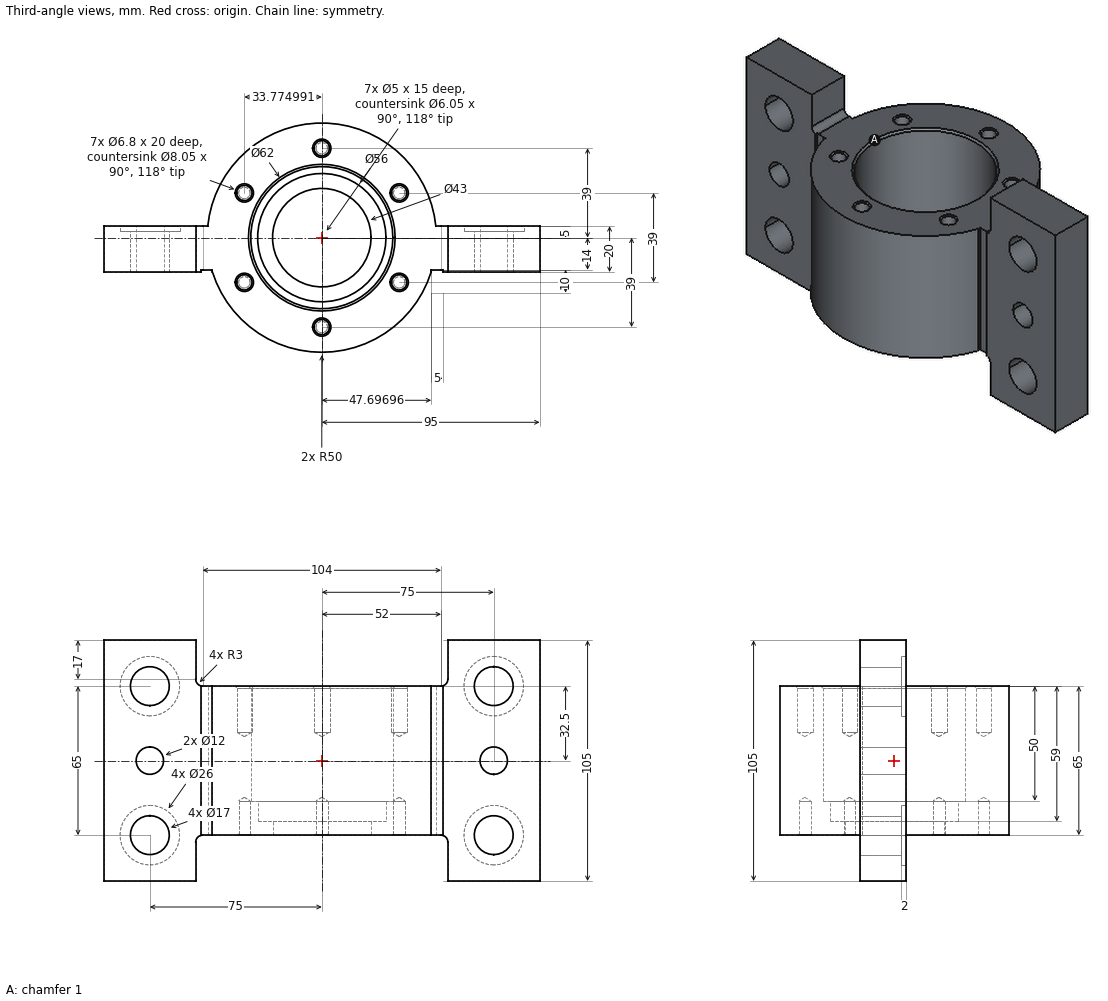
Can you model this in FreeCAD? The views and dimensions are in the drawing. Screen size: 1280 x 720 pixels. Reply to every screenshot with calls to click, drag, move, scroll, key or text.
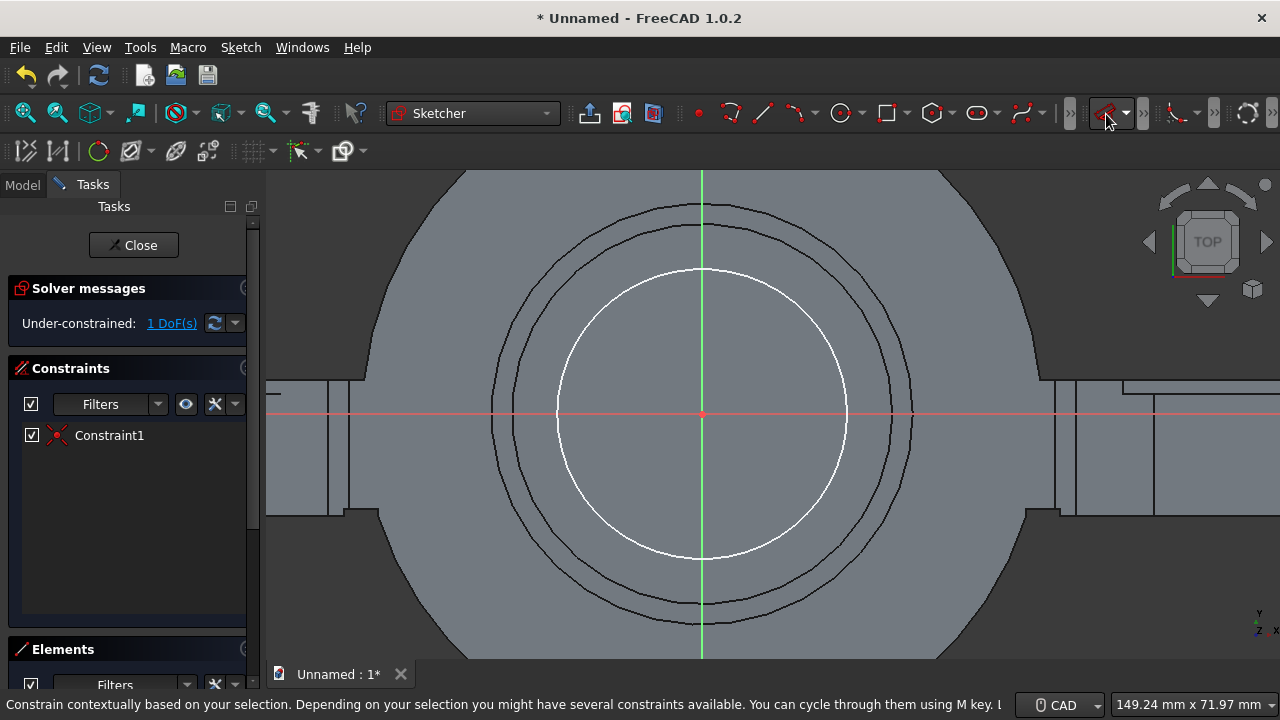
click(804, 311)
click(826, 288)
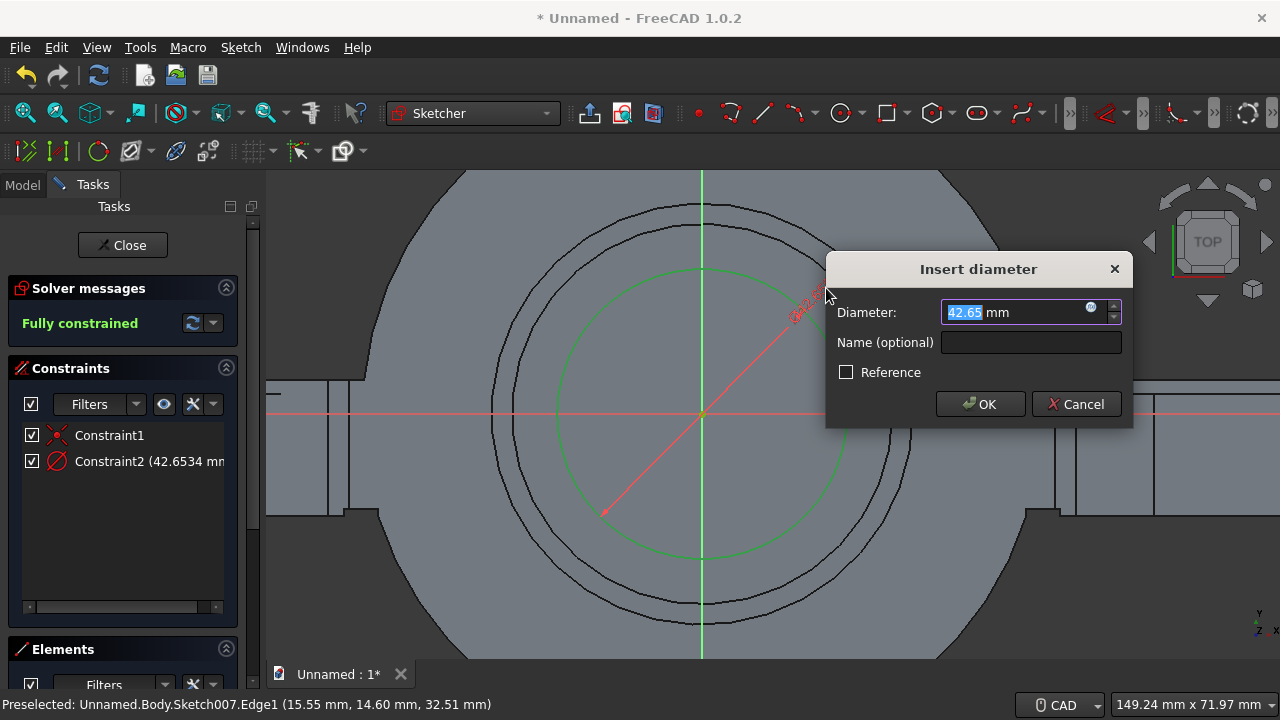
text(43)
key(Return)
key(Escape)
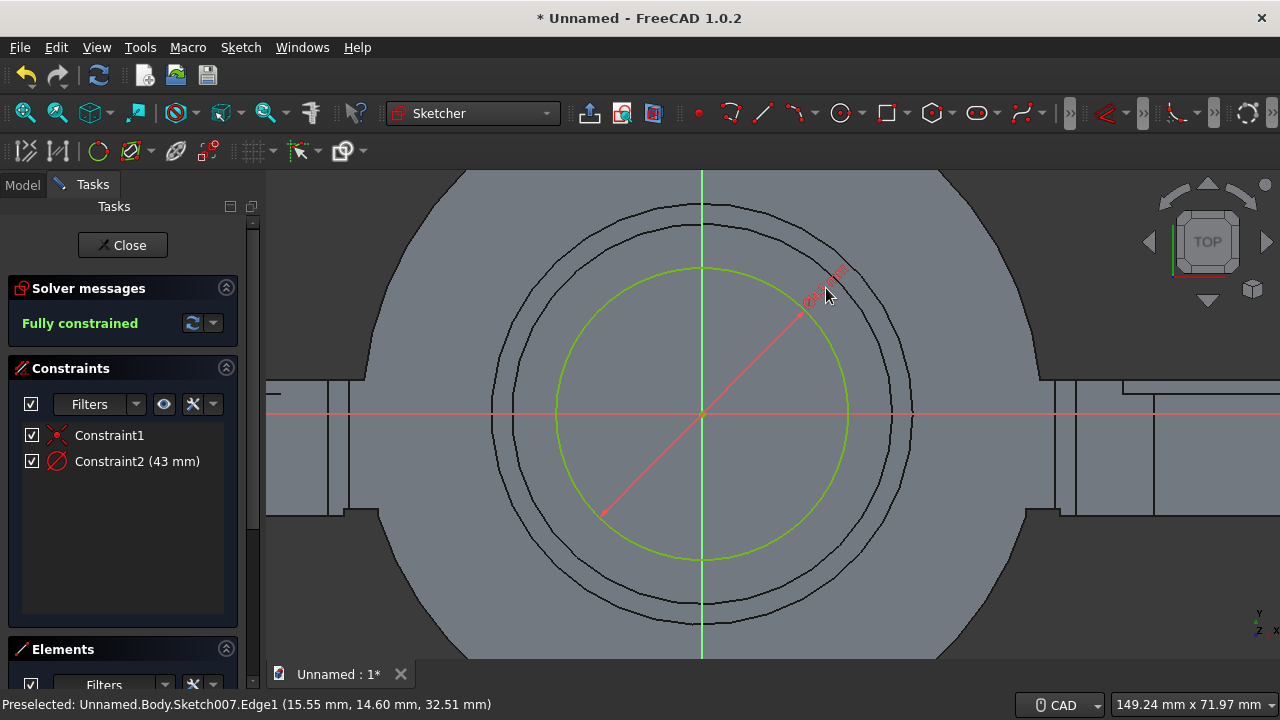
click(123, 245)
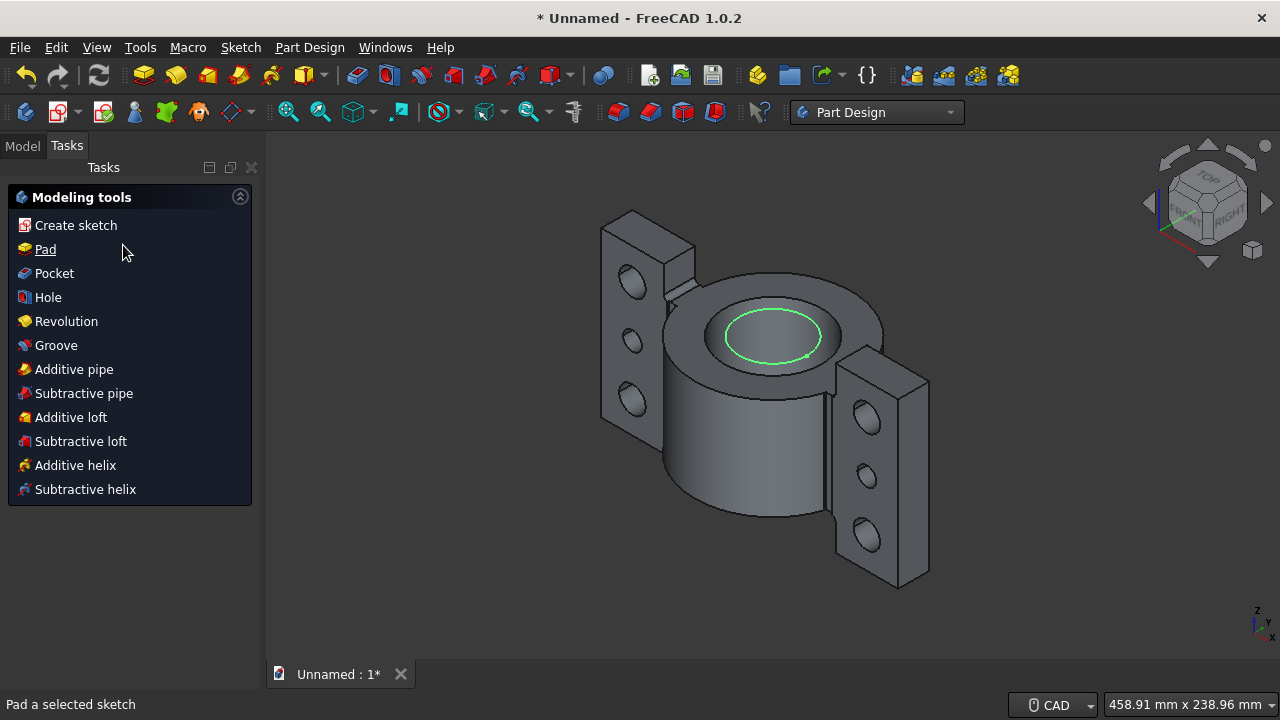
click(358, 76)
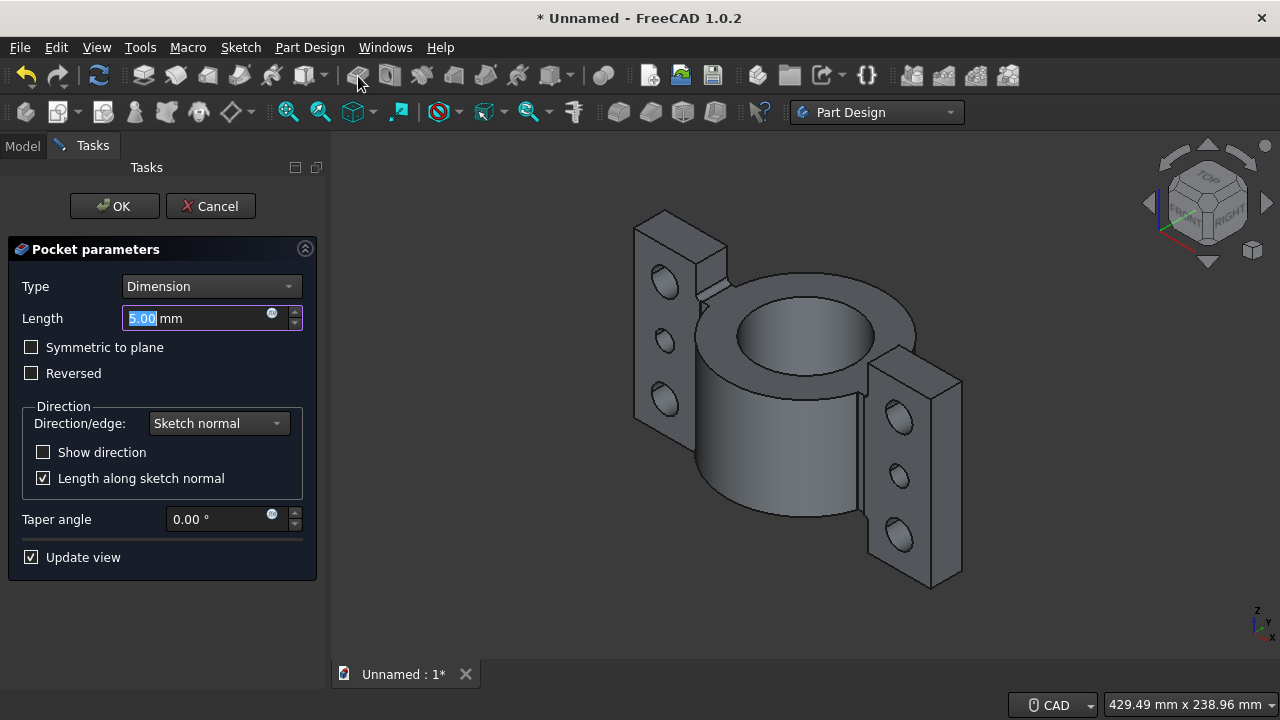
text(65)
key(Tab)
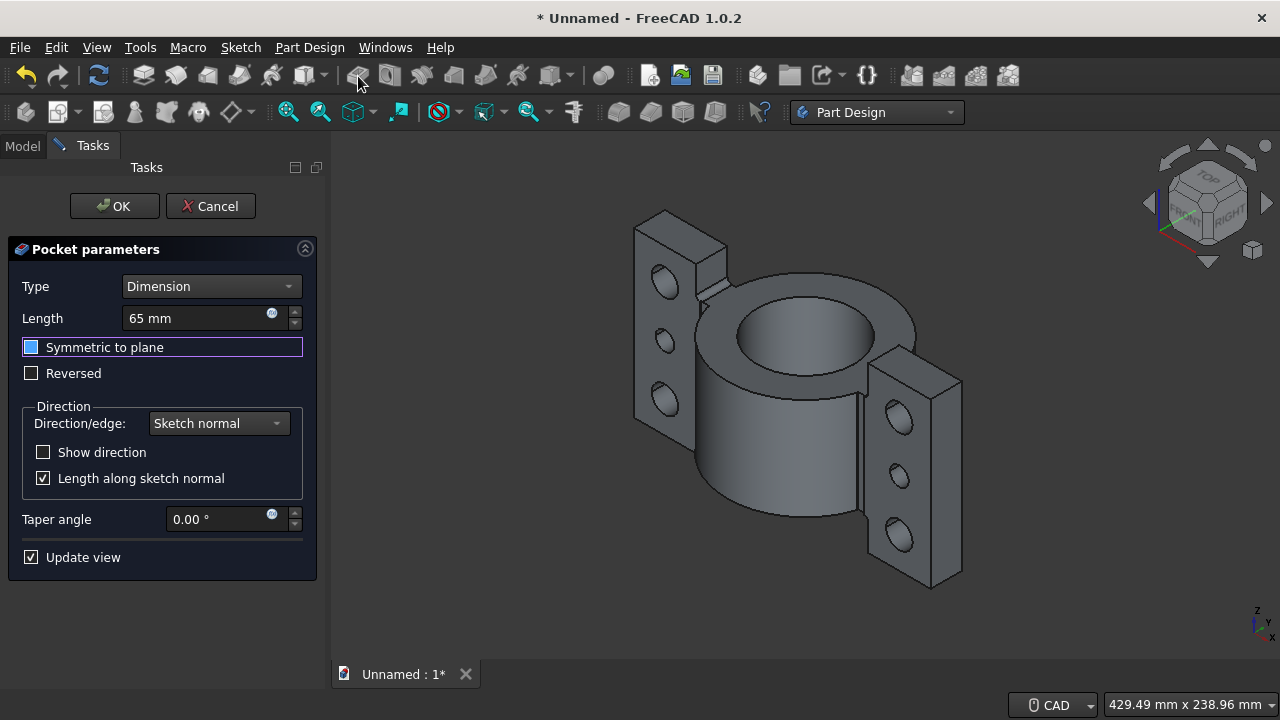
click(115, 206)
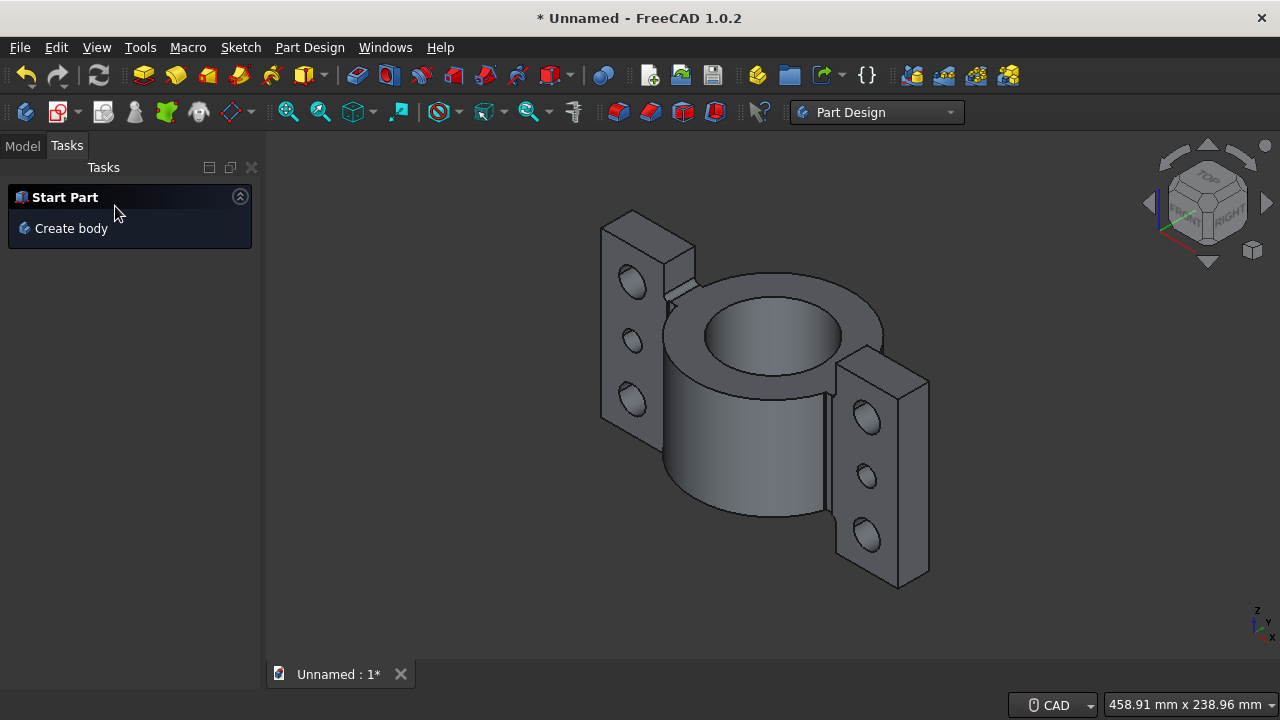
click(725, 307)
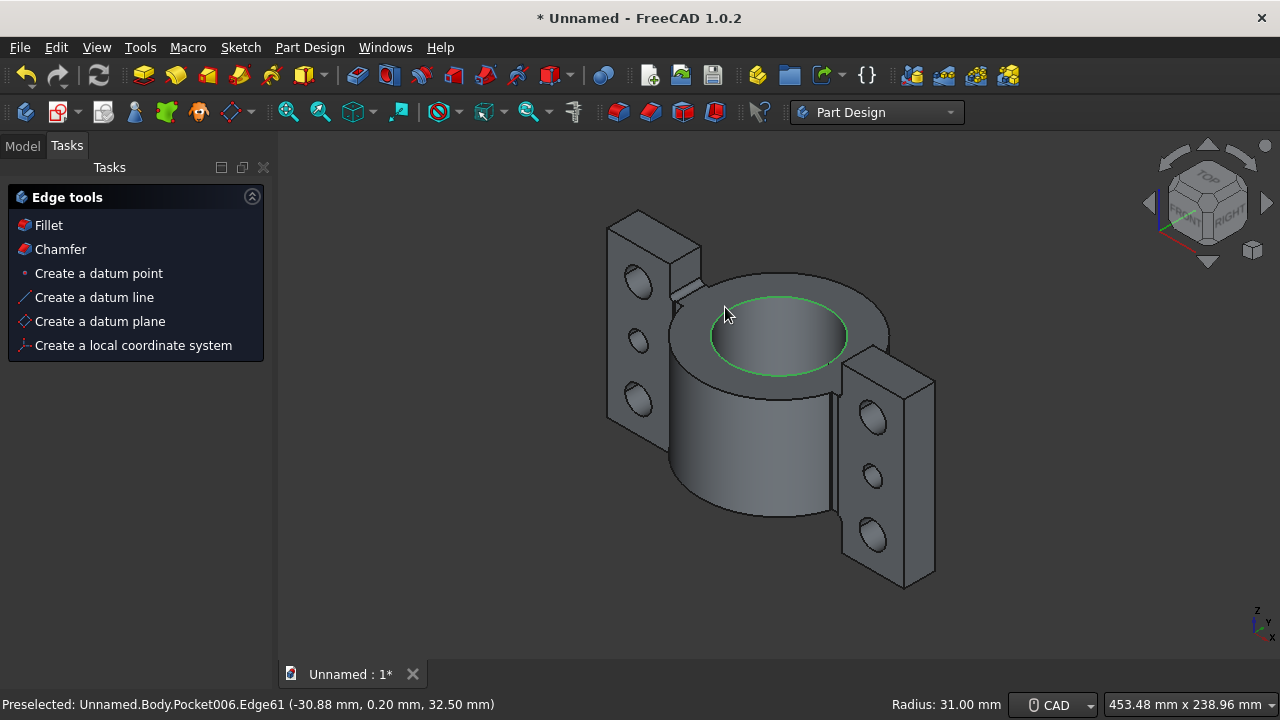
click(652, 112)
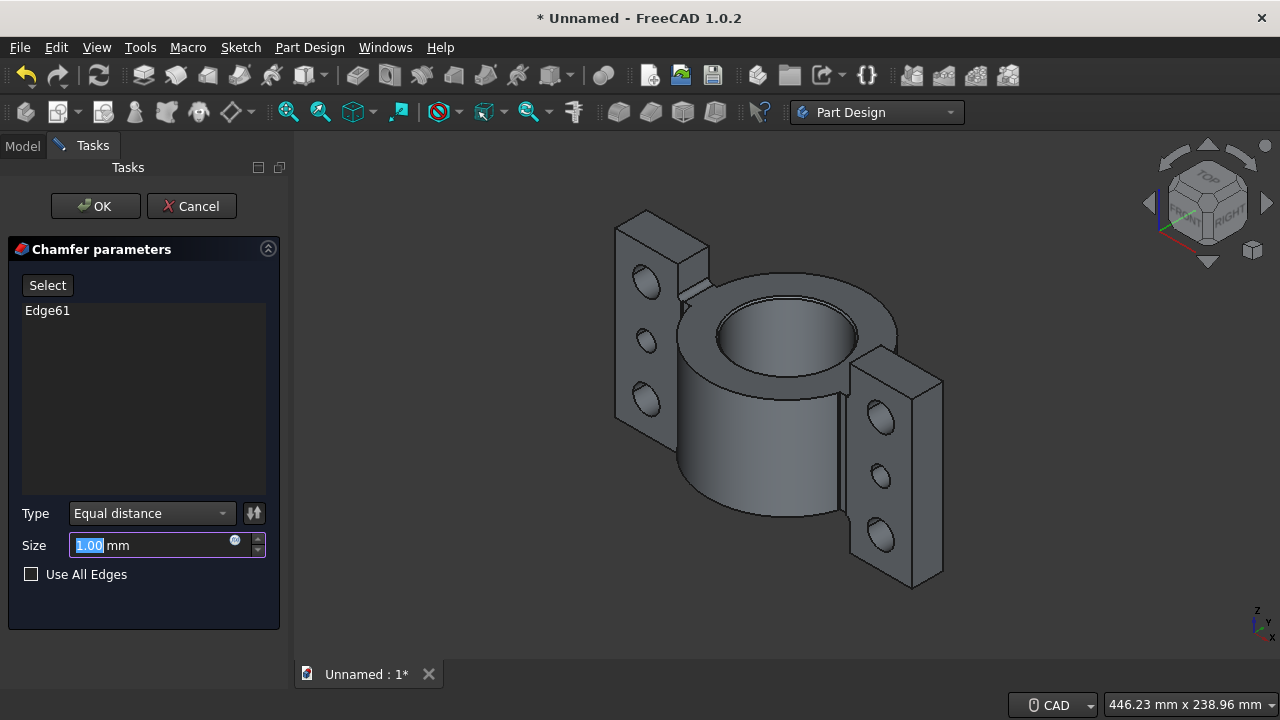
text(1)
key(Tab)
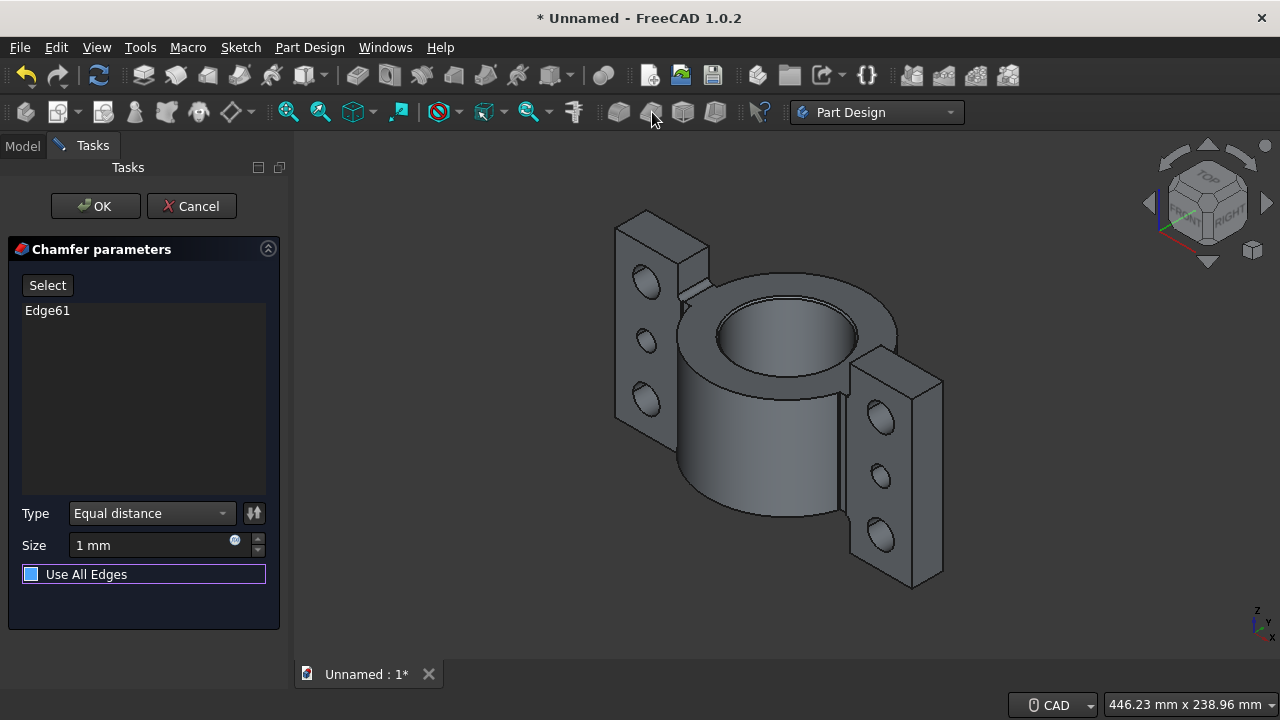
click(96, 206)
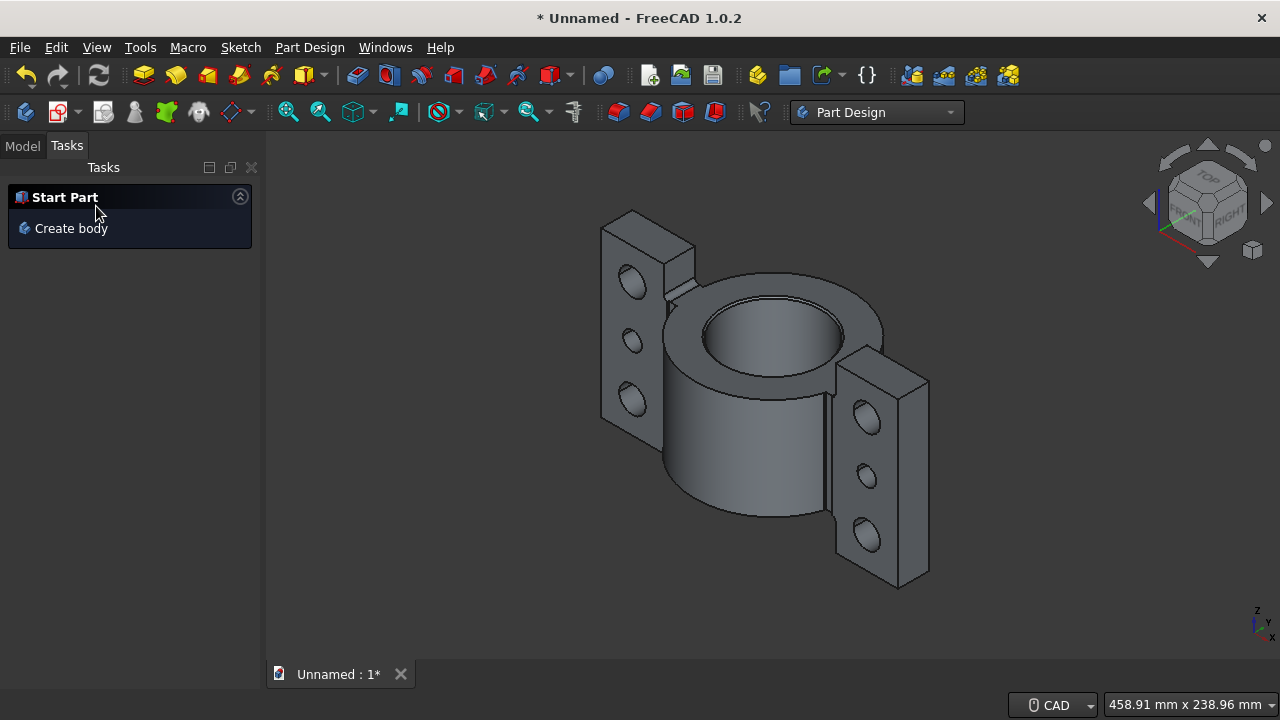
click(771, 283)